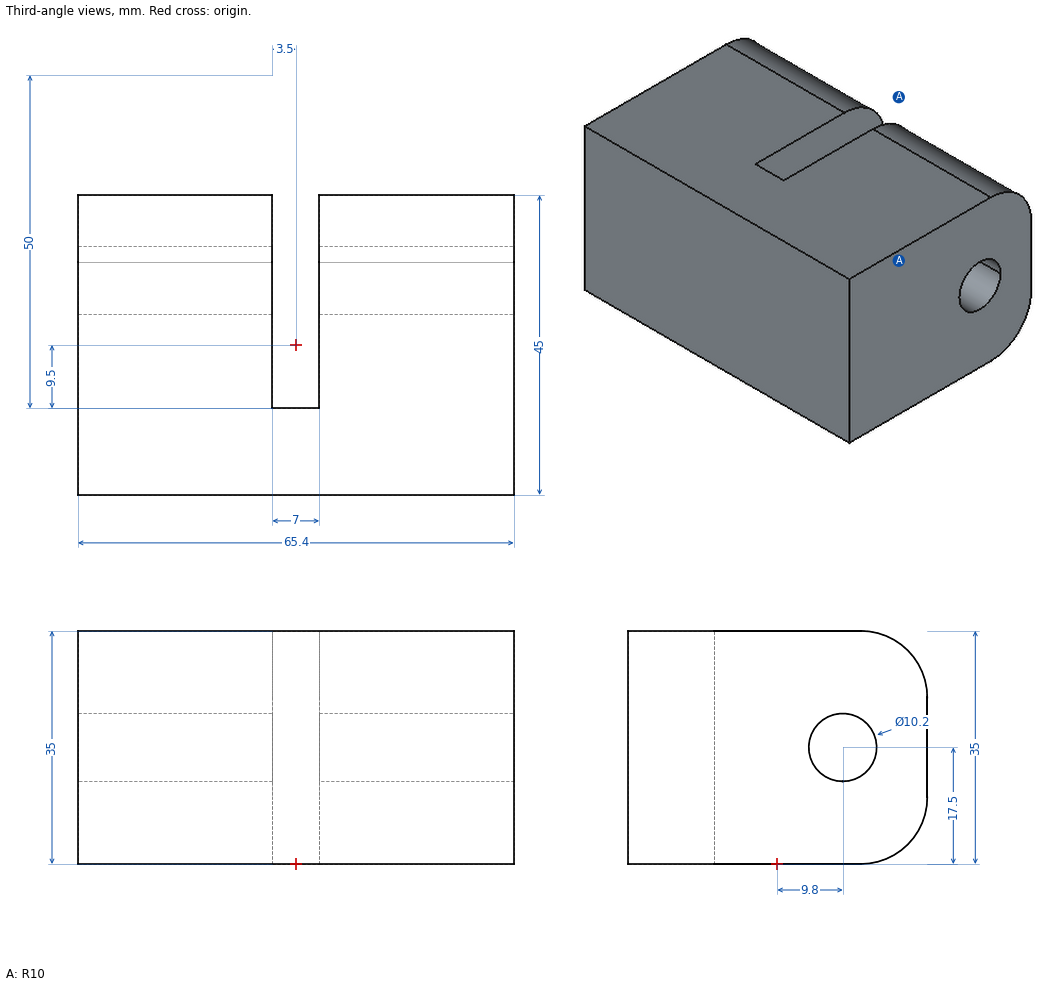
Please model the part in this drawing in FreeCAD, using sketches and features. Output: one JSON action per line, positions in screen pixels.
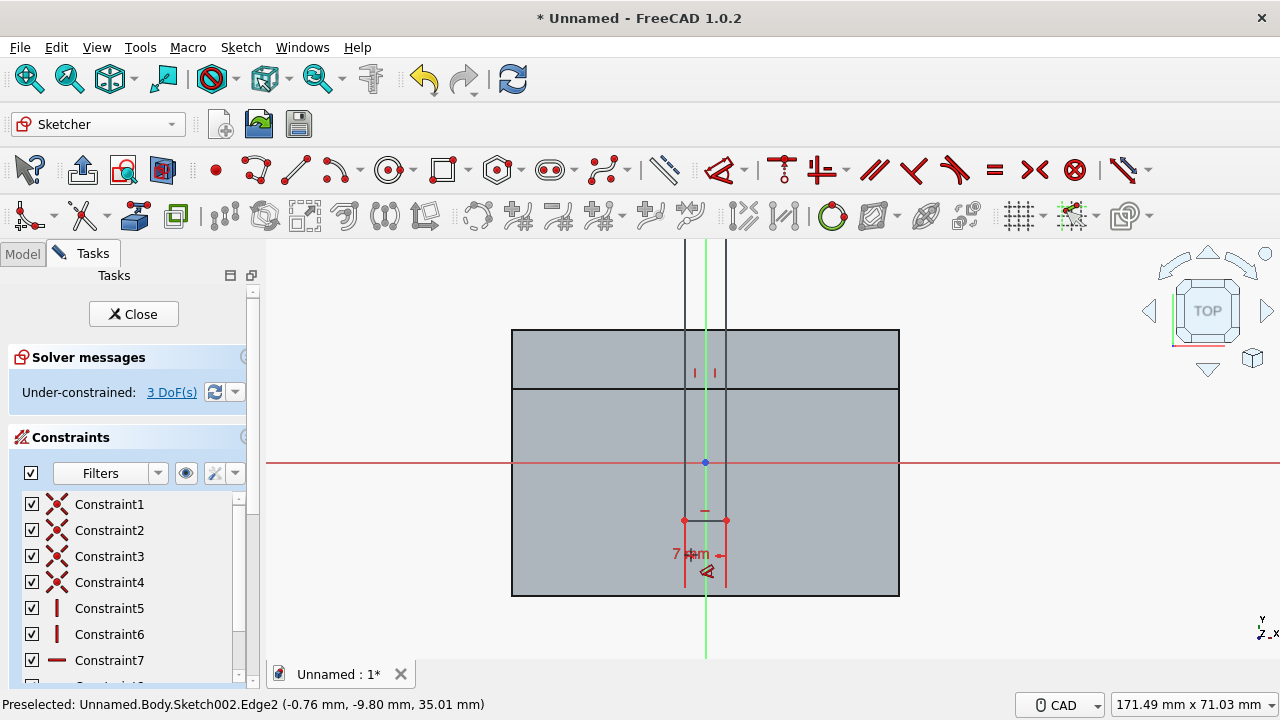
{"action": "left_click", "coordinate": [685, 314]}
{"action": "left_click", "coordinate": [651, 394]}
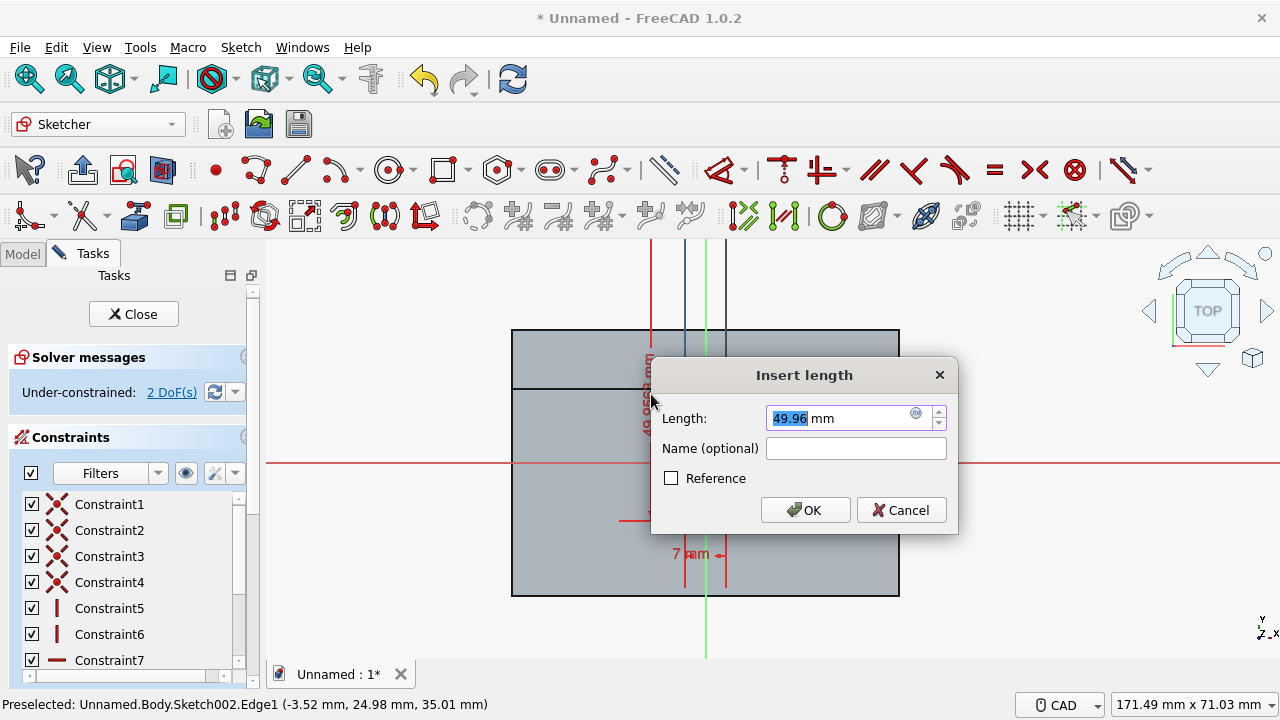
{"action": "type", "text": "50"}
{"action": "key", "text": "Return"}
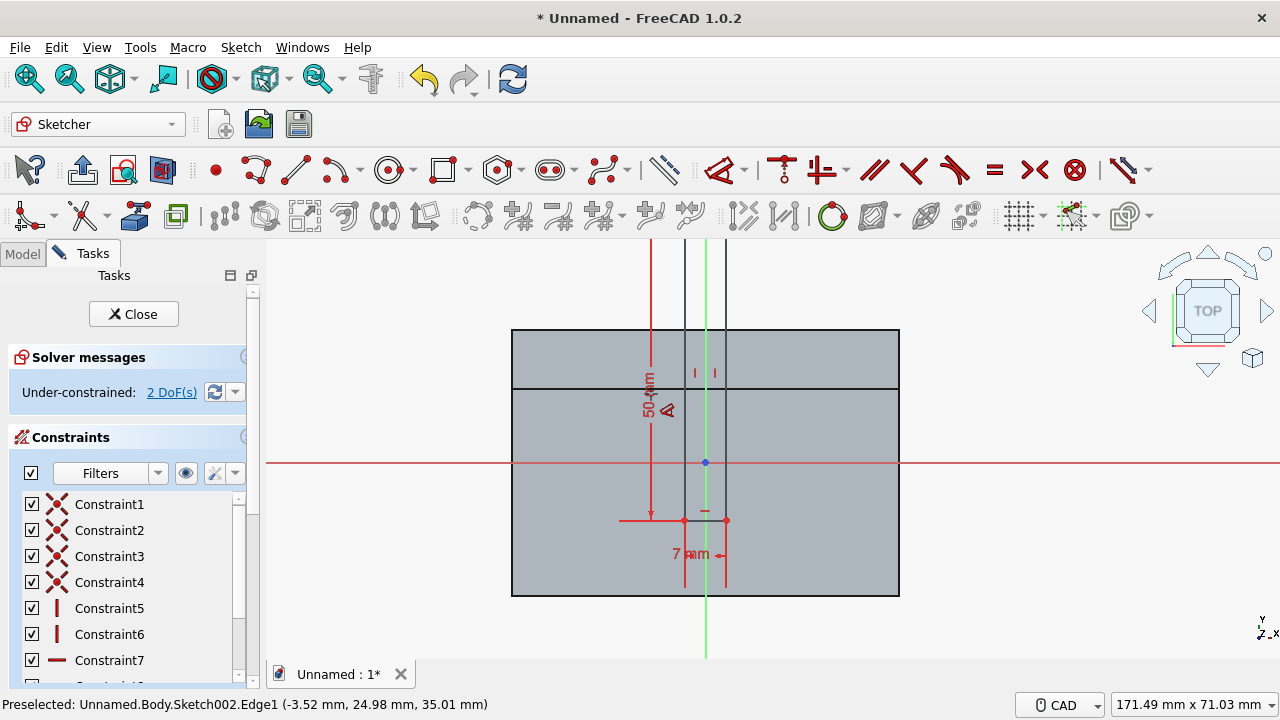
{"action": "scroll", "coordinate": [700, 631], "scroll_direction": "down", "scroll_amount": 1}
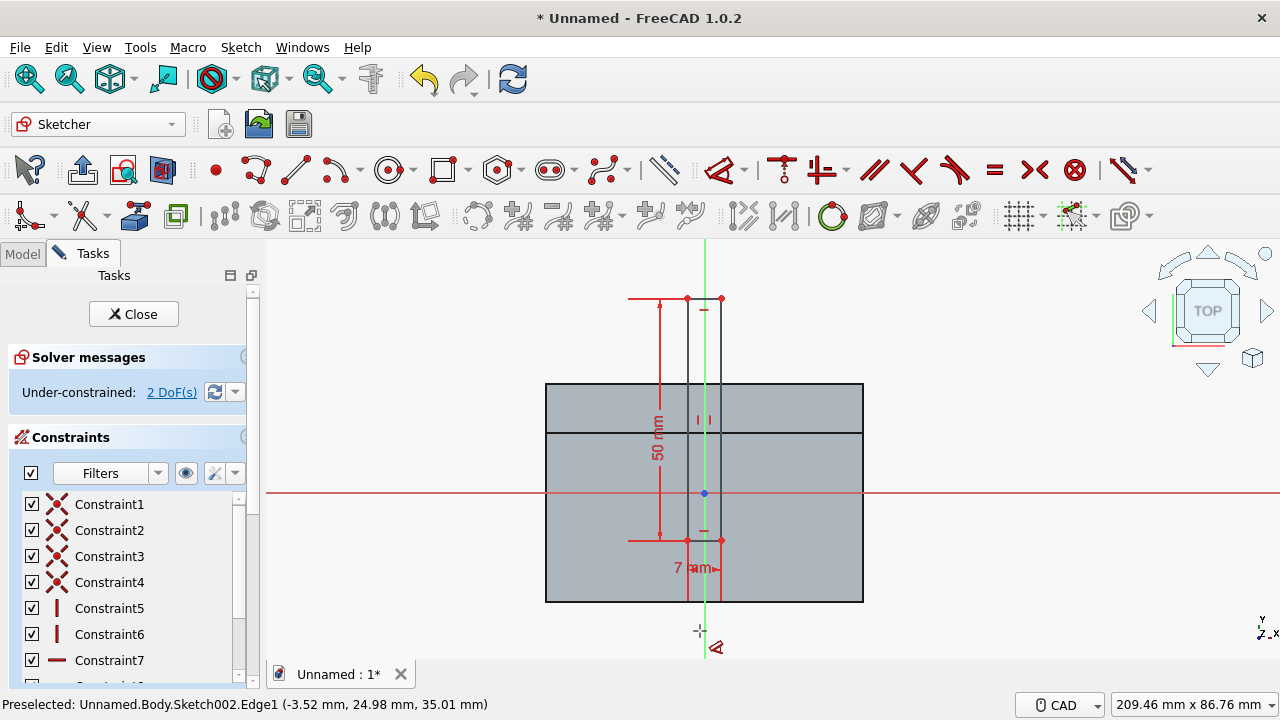
{"action": "scroll", "coordinate": [688, 299], "scroll_direction": "up", "scroll_amount": 5}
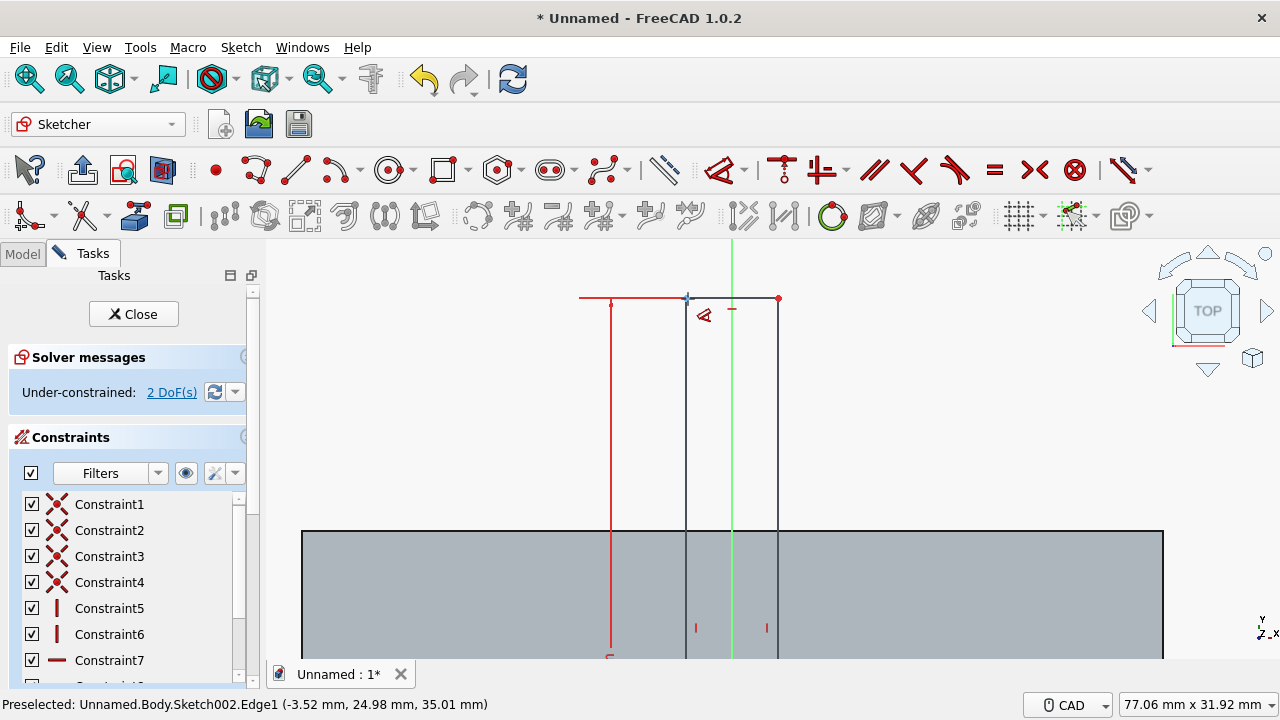
{"action": "left_click", "coordinate": [686, 298]}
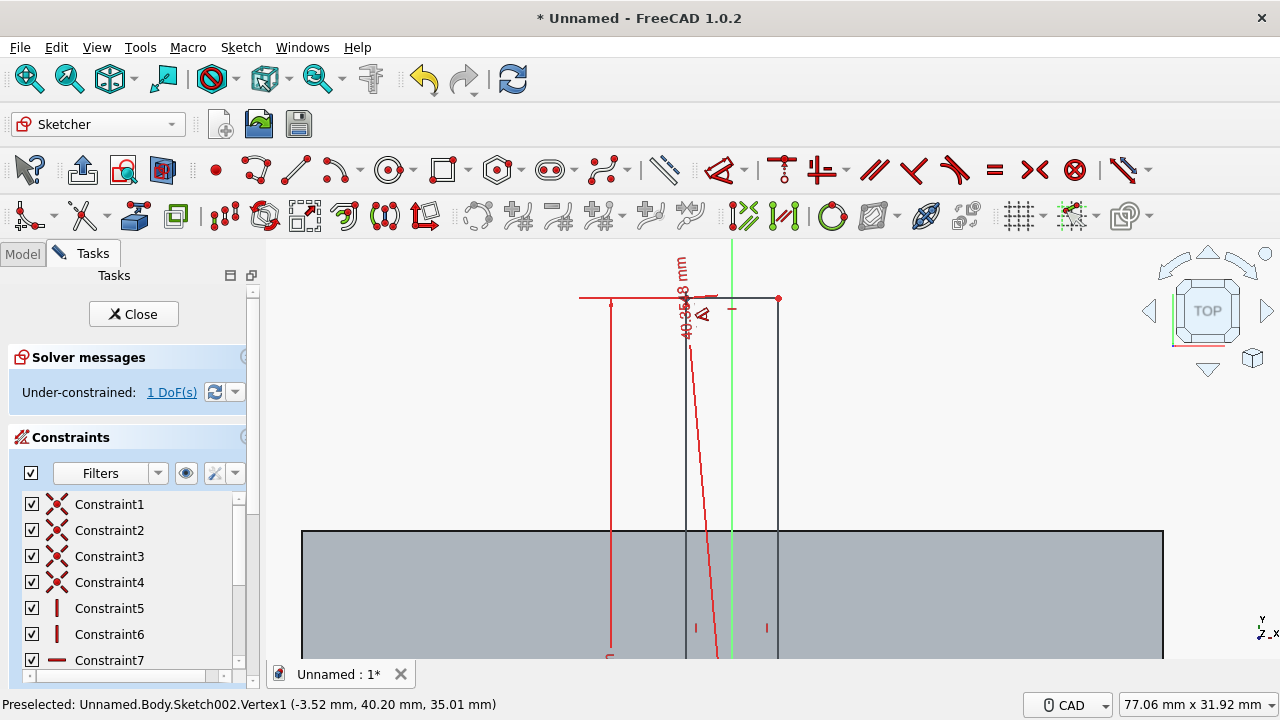
{"action": "key", "text": "Escape"}
{"action": "key", "text": "Escape"}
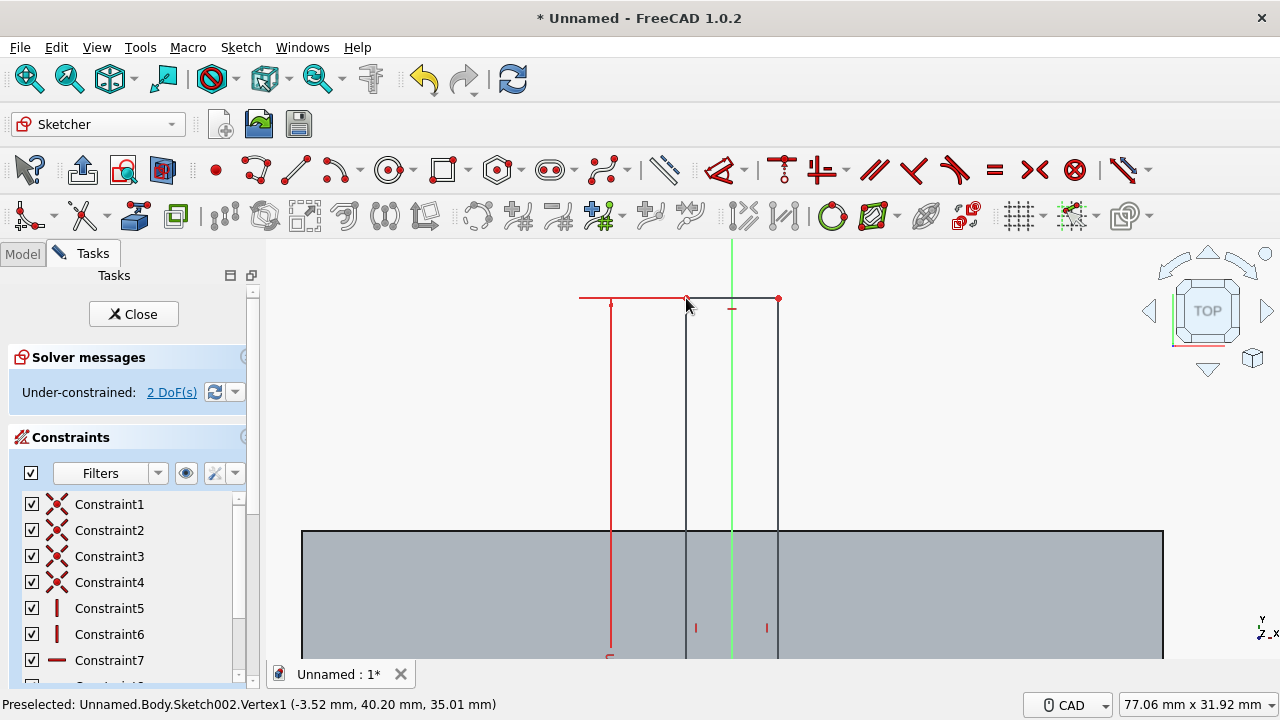
{"action": "left_click", "coordinate": [686, 298]}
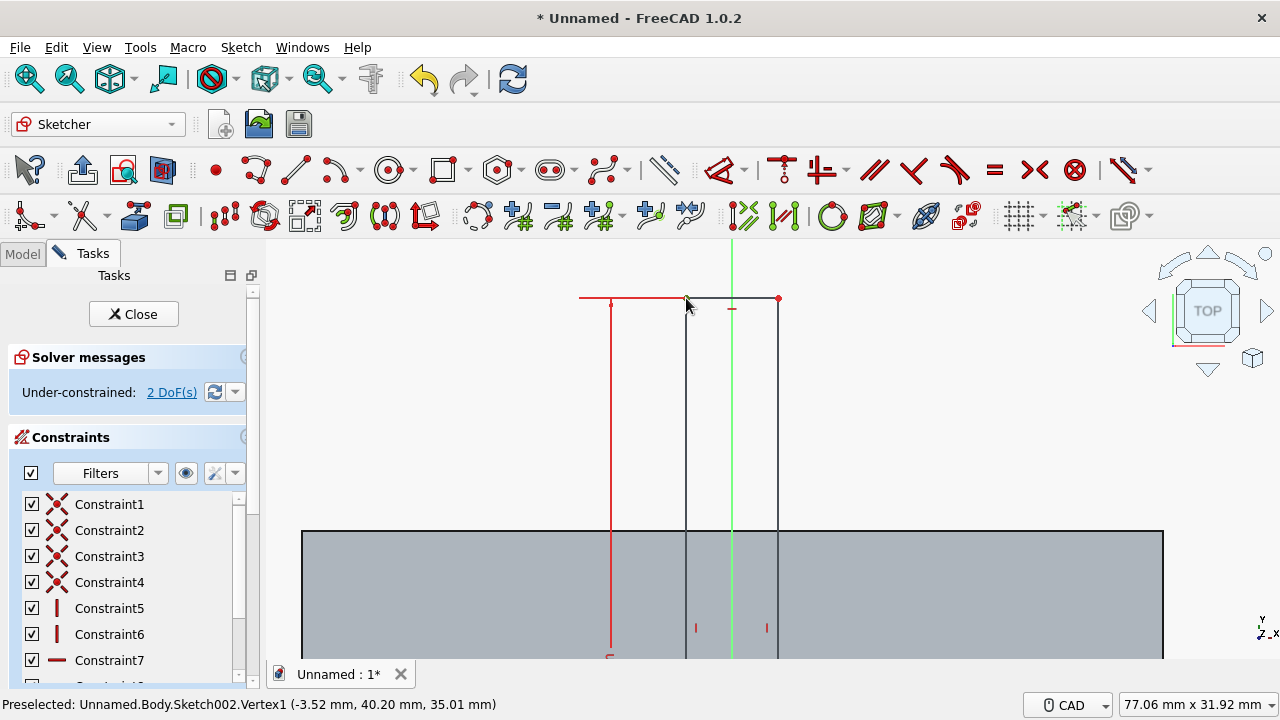
{"action": "left_click", "coordinate": [746, 170]}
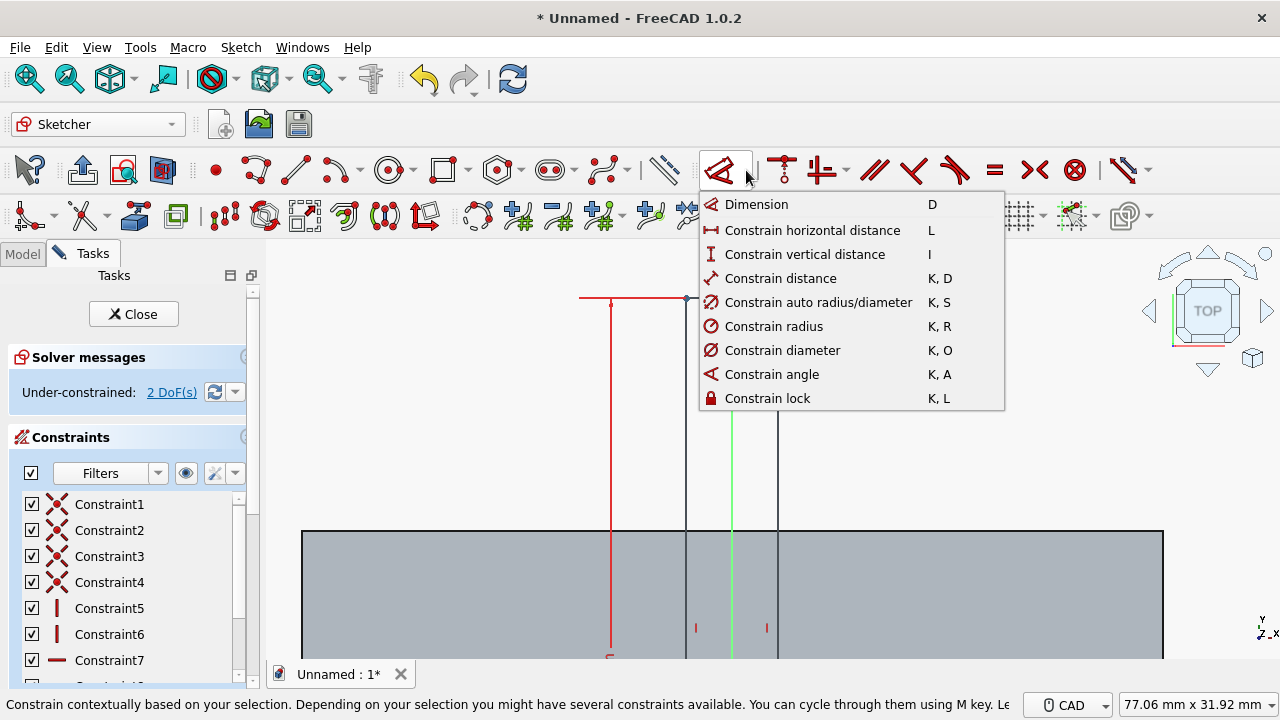
{"action": "left_click", "coordinate": [852, 230]}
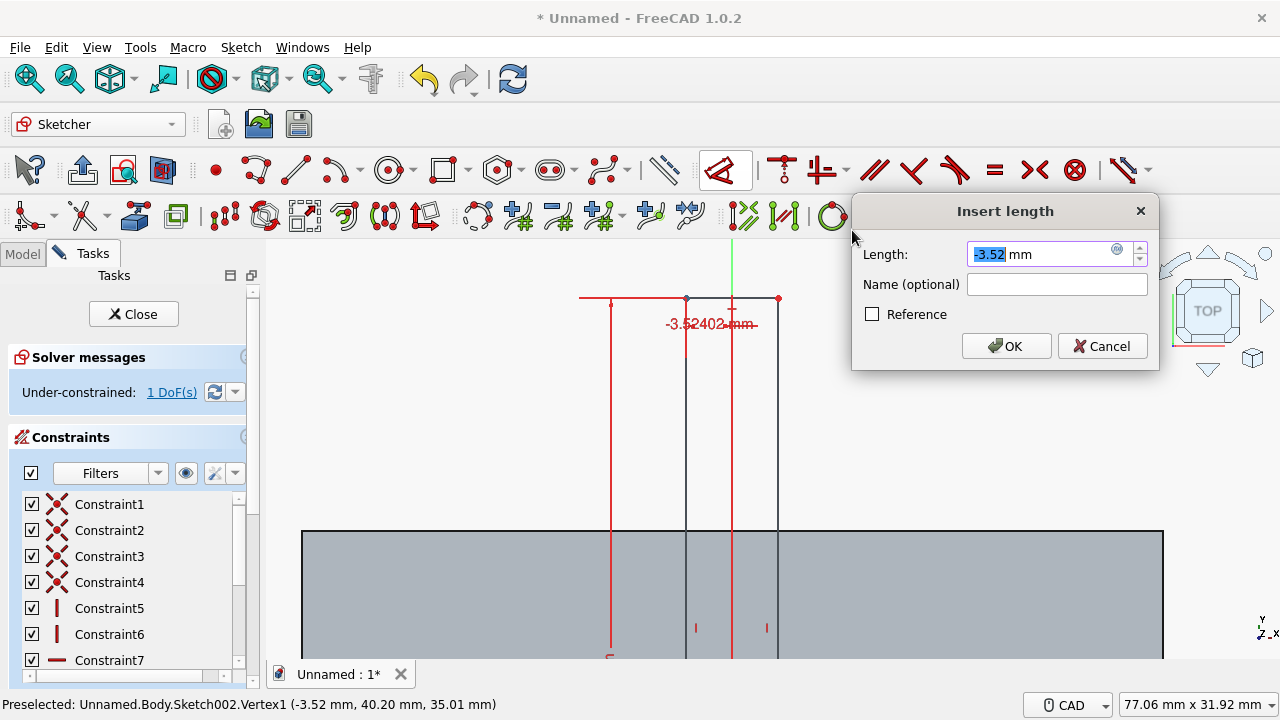
{"action": "type", "text": "-3.5"}
{"action": "key", "text": "Return"}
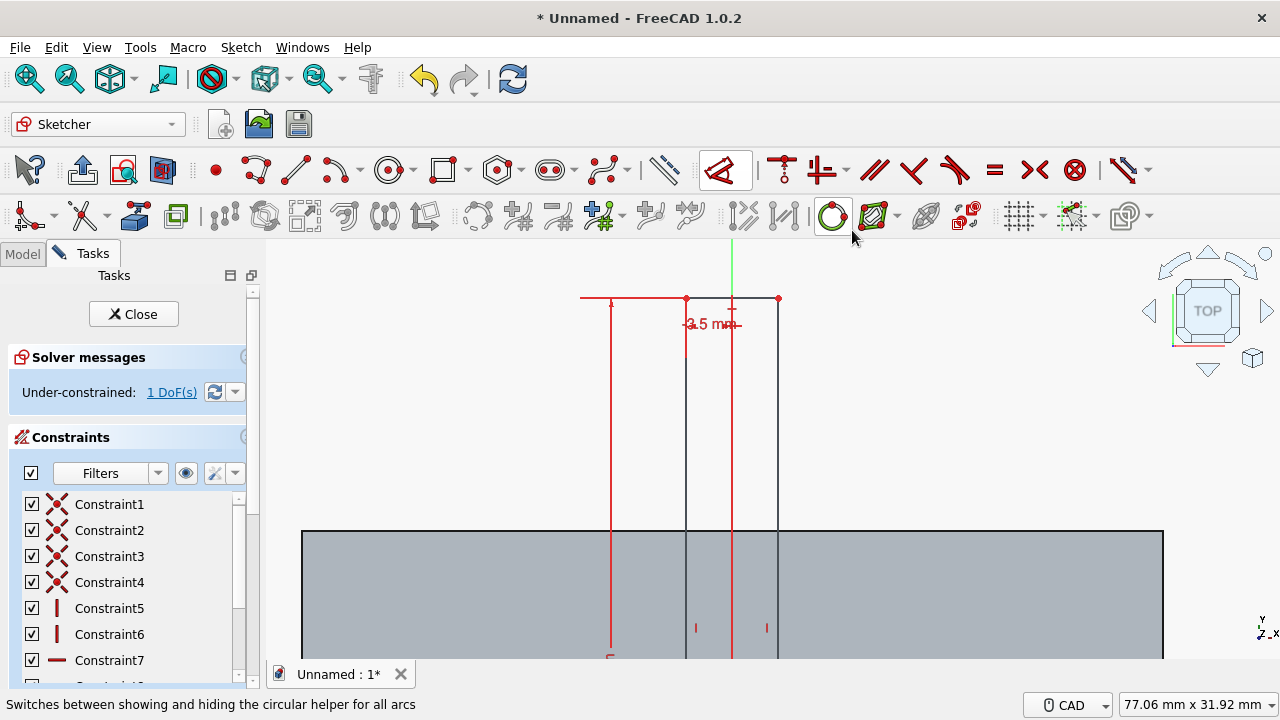
{"action": "scroll", "coordinate": [688, 348], "scroll_direction": "down", "scroll_amount": 5}